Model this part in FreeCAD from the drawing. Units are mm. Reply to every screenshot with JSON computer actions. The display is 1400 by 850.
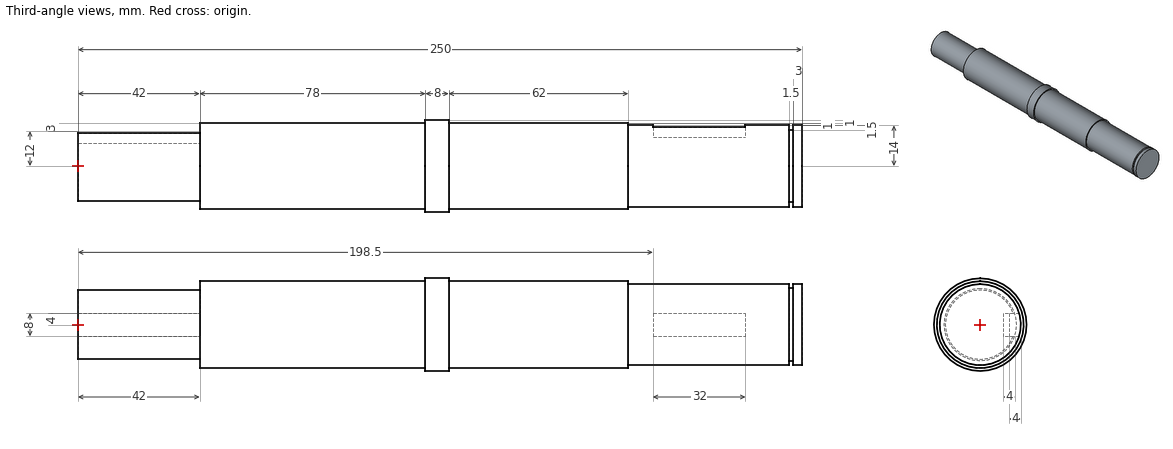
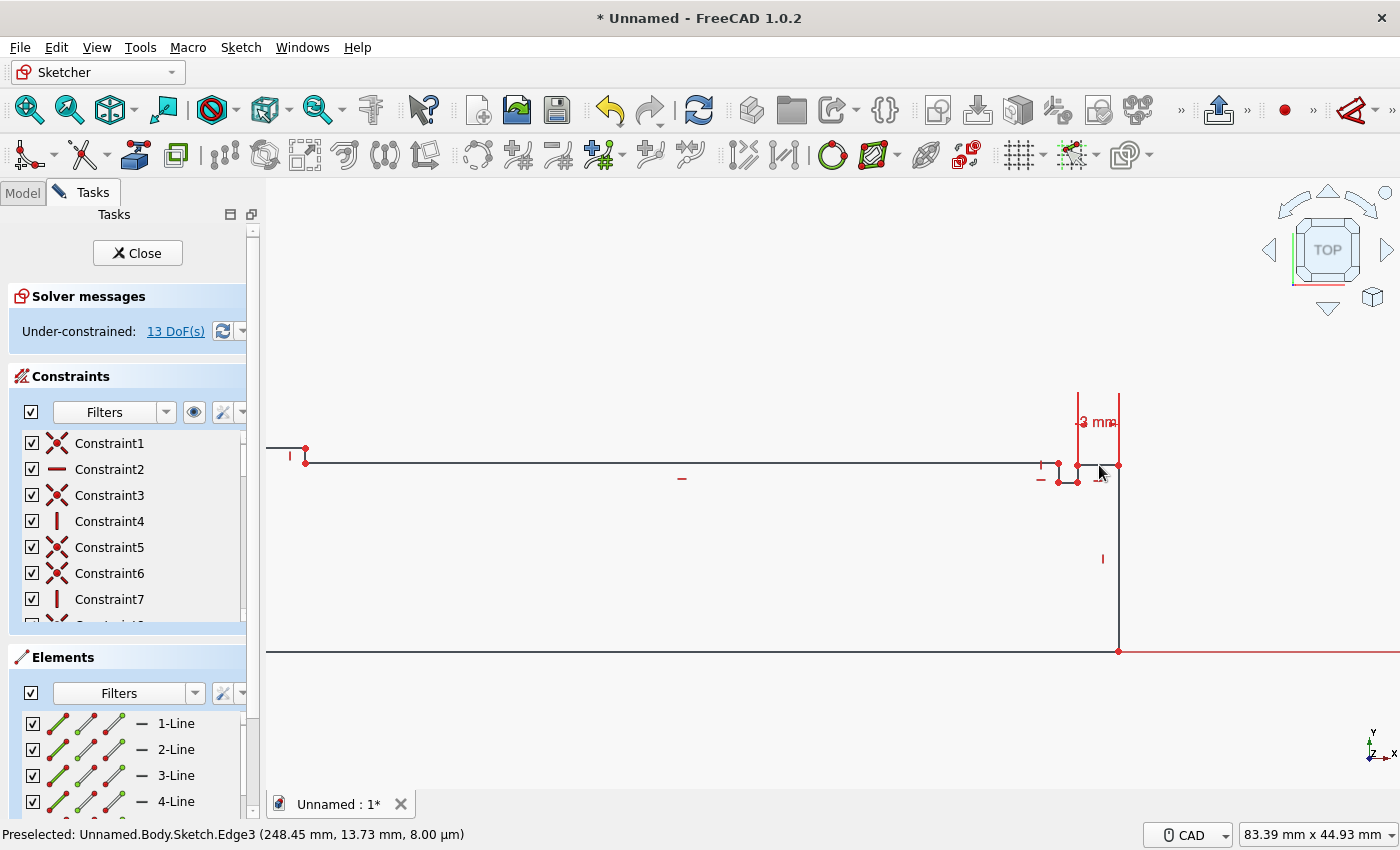
{"action": "scroll", "coordinate": [305, 456], "scroll_direction": "up", "scroll_amount": 6}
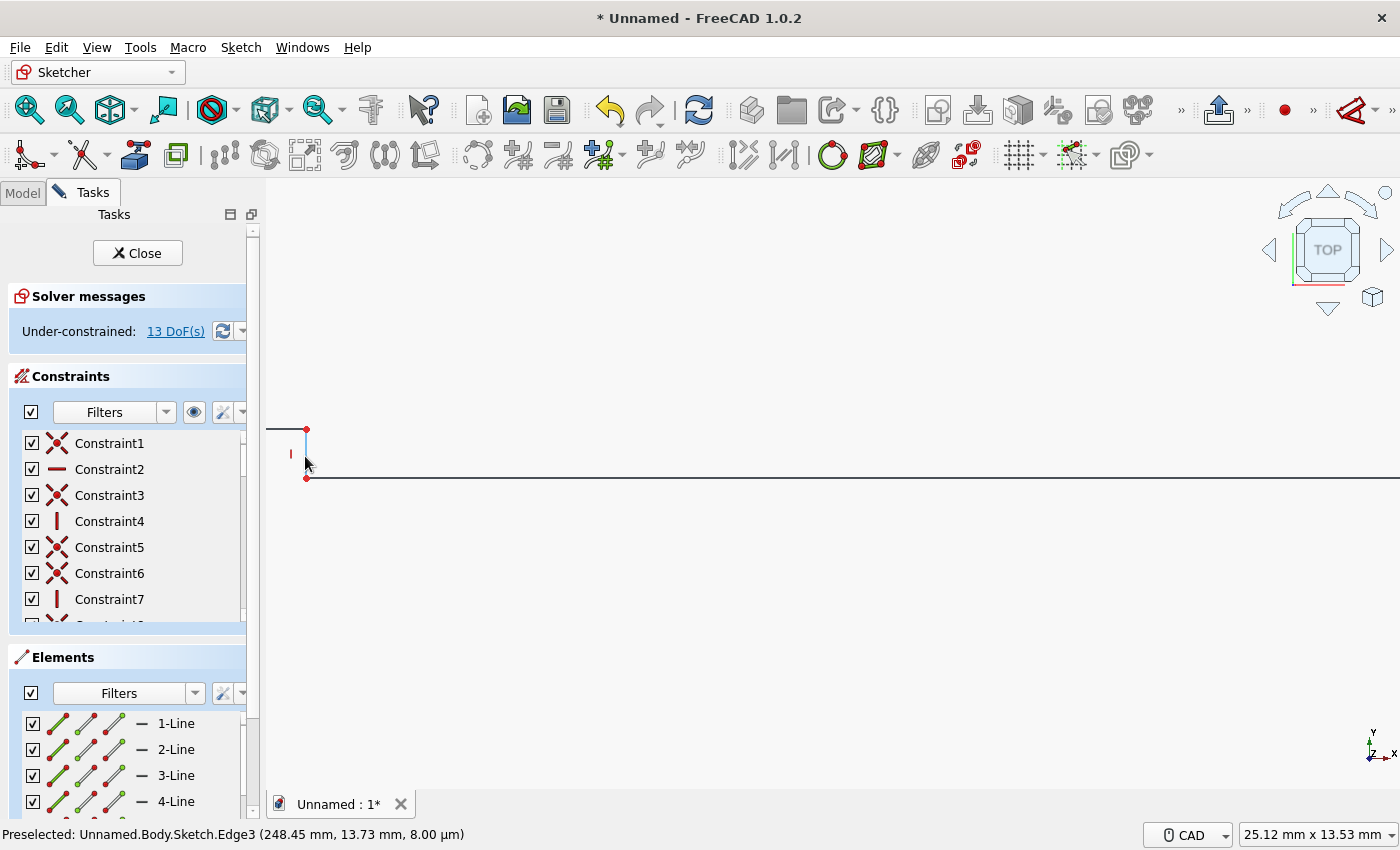
{"action": "left_click", "coordinate": [306, 454]}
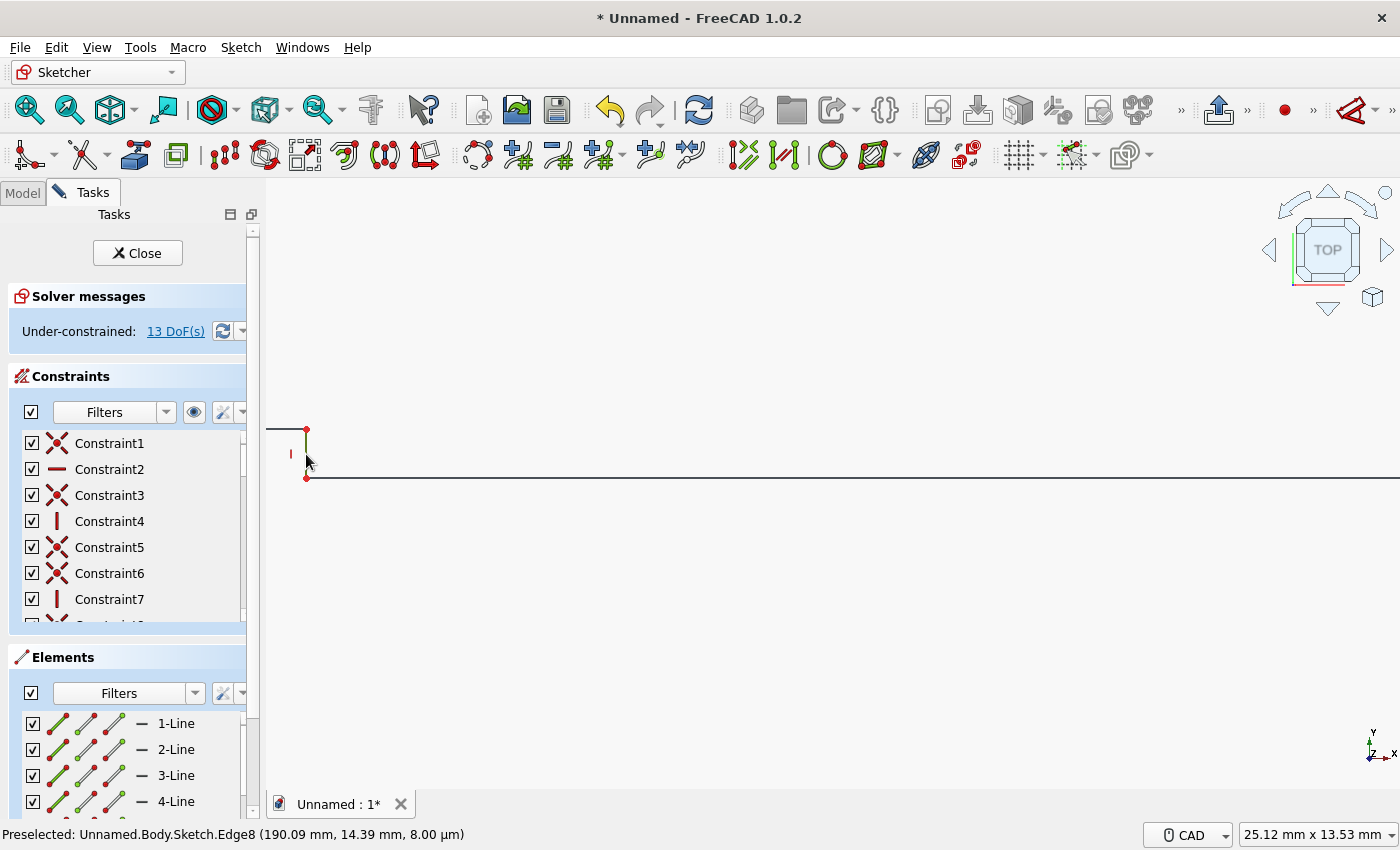
{"action": "left_click", "coordinate": [1378, 110]}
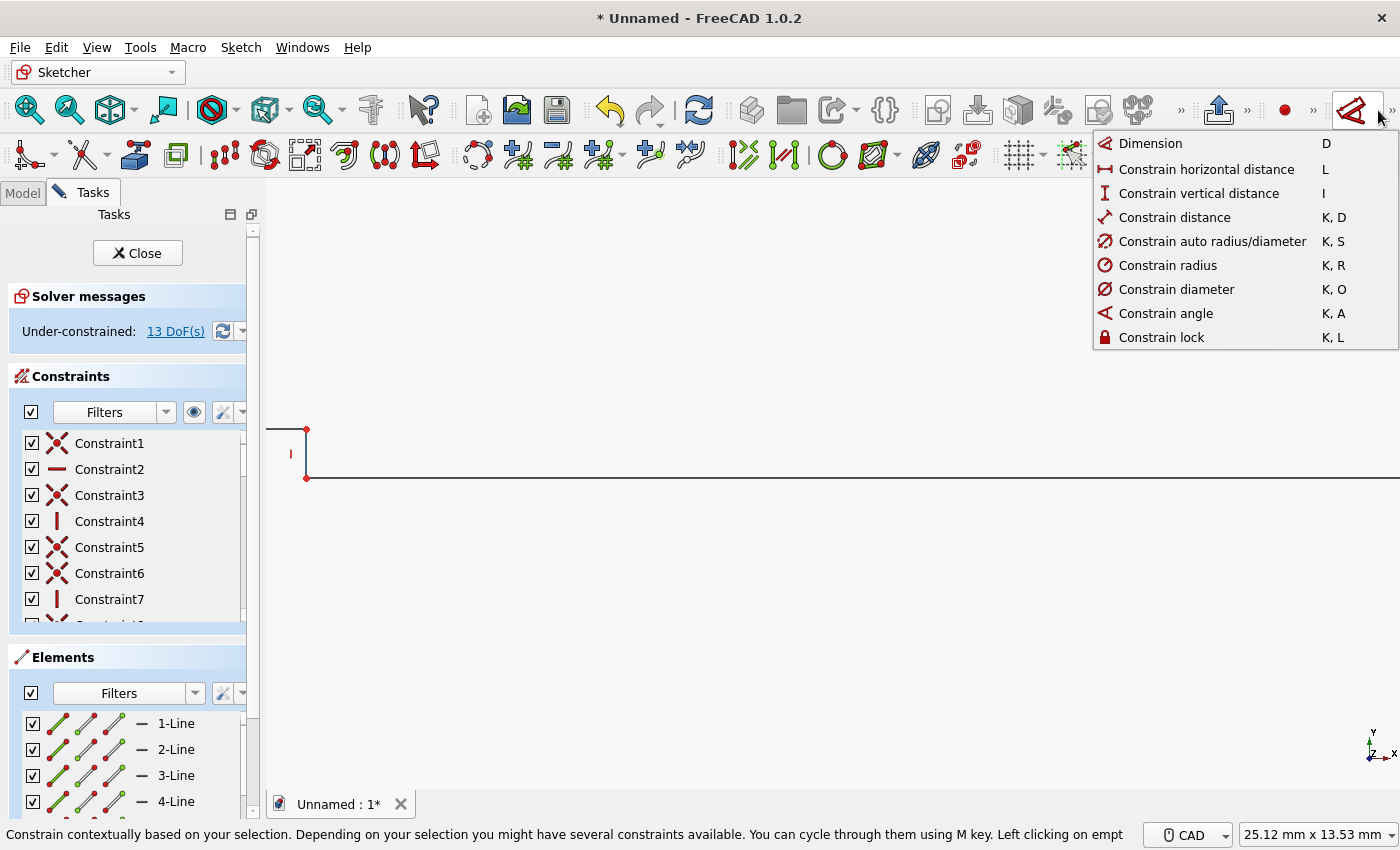
{"action": "left_click", "coordinate": [1246, 193]}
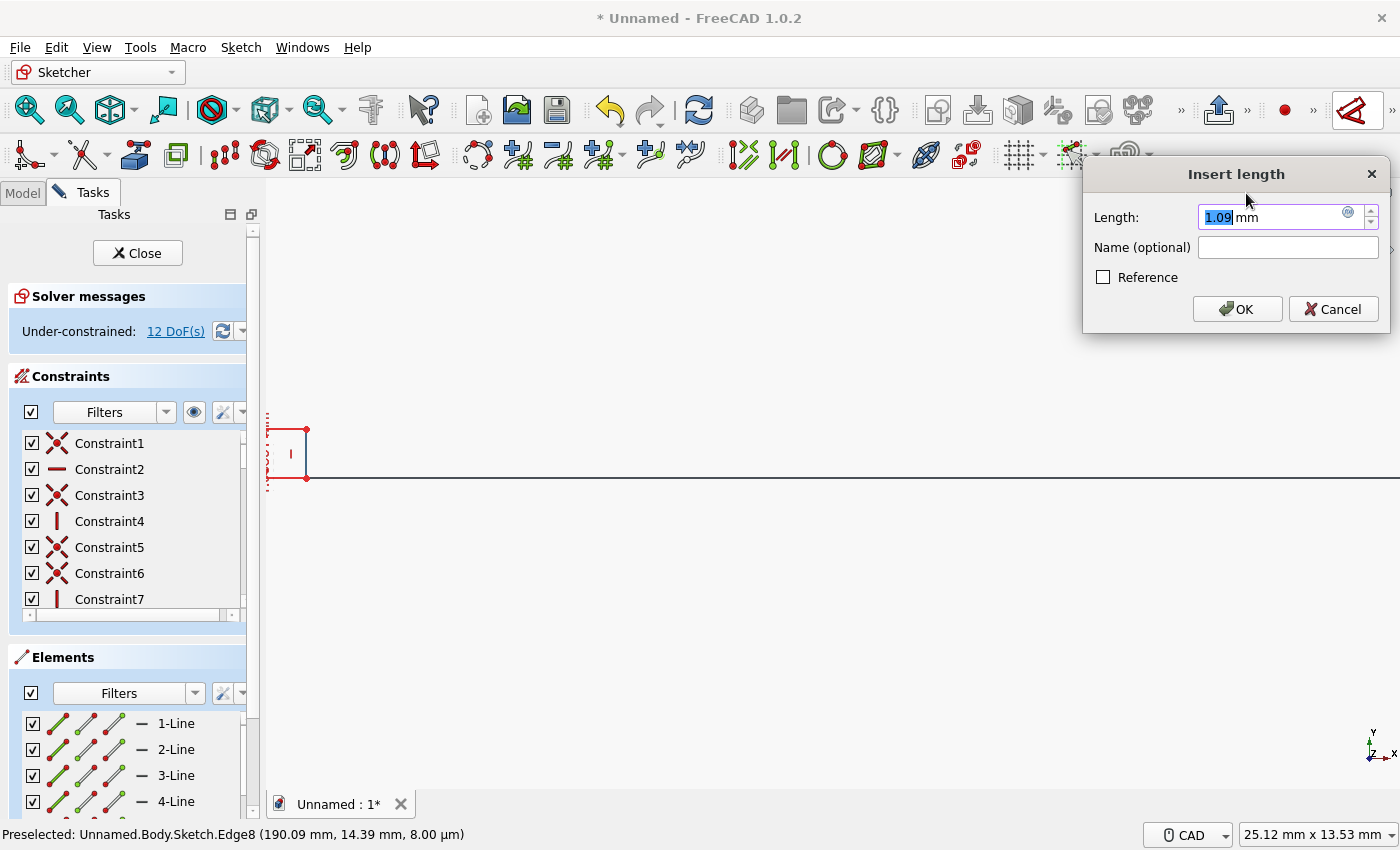
{"action": "type", "text": "1"}
{"action": "key", "text": "Return"}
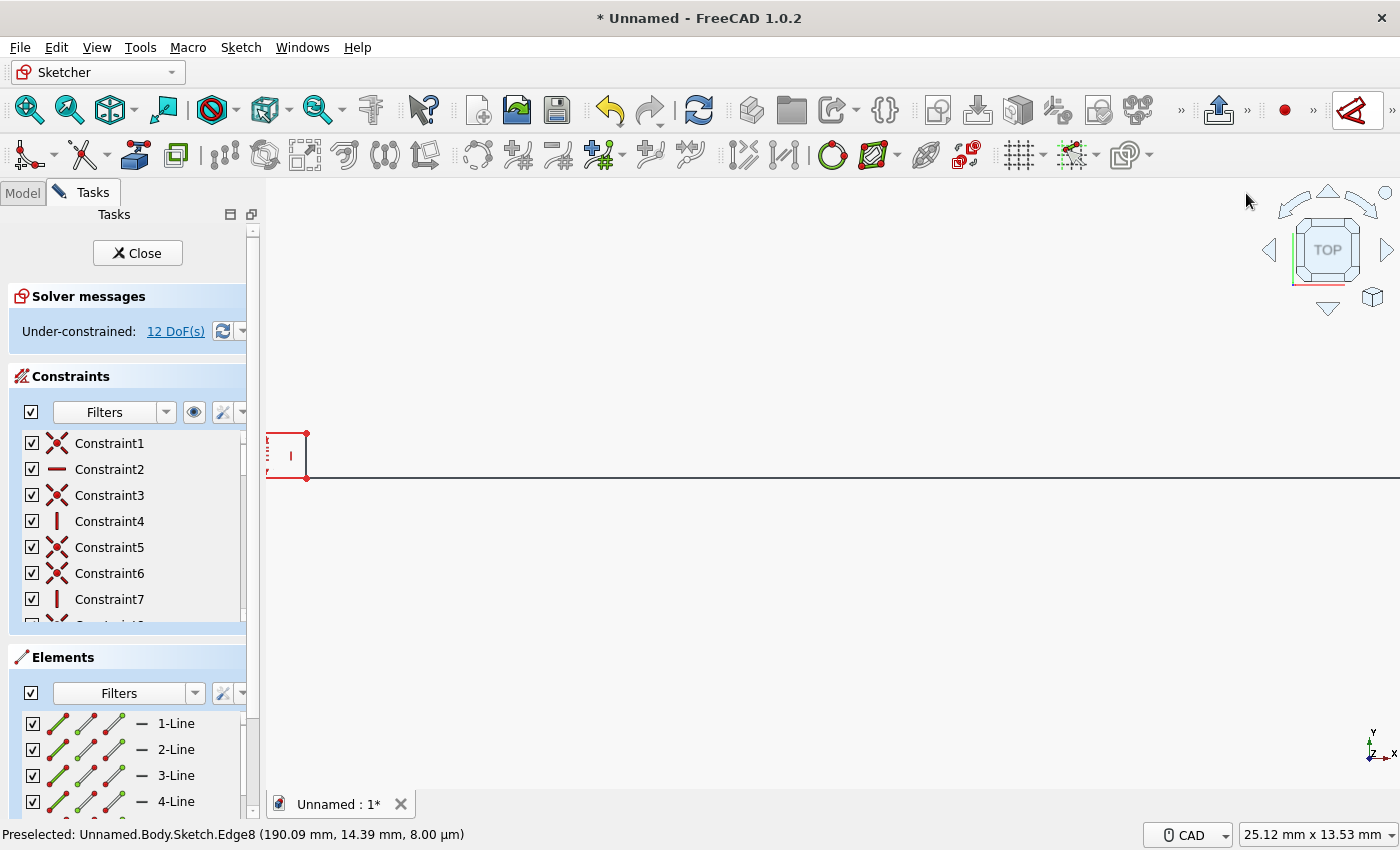
{"action": "scroll", "coordinate": [984, 467], "scroll_direction": "down", "scroll_amount": 14}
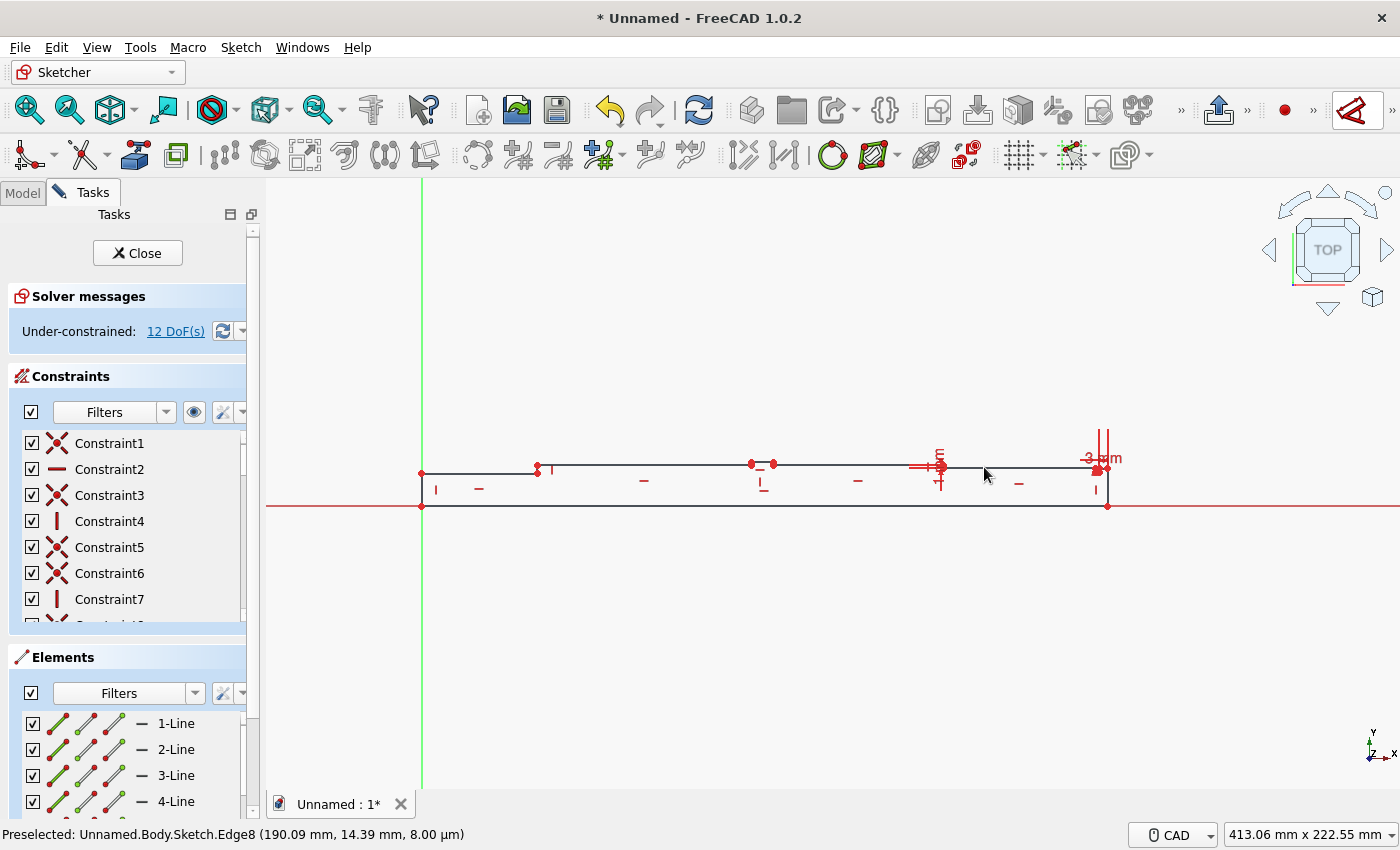
{"action": "scroll", "coordinate": [773, 465], "scroll_direction": "up", "scroll_amount": 14}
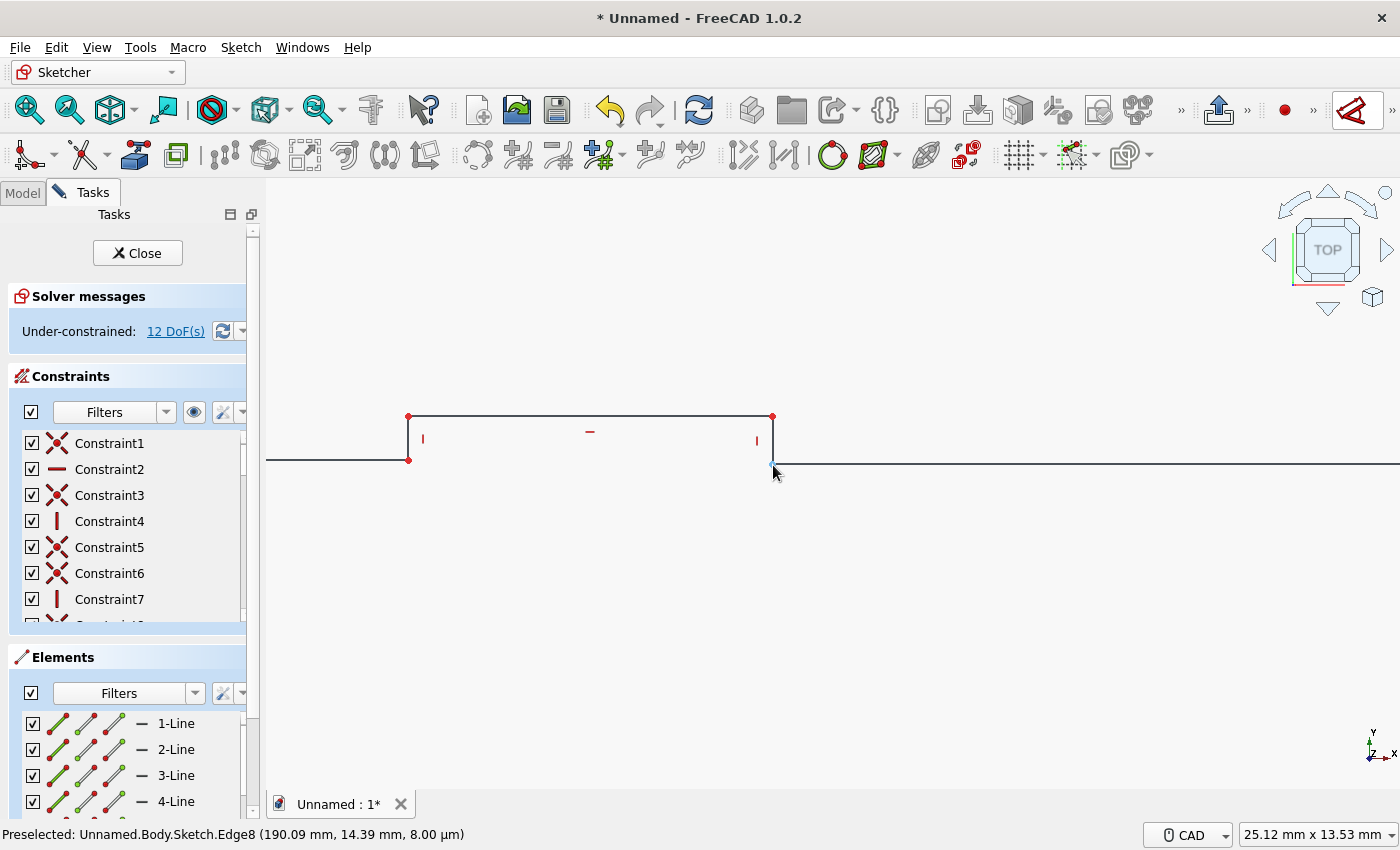
{"action": "left_click", "coordinate": [773, 450]}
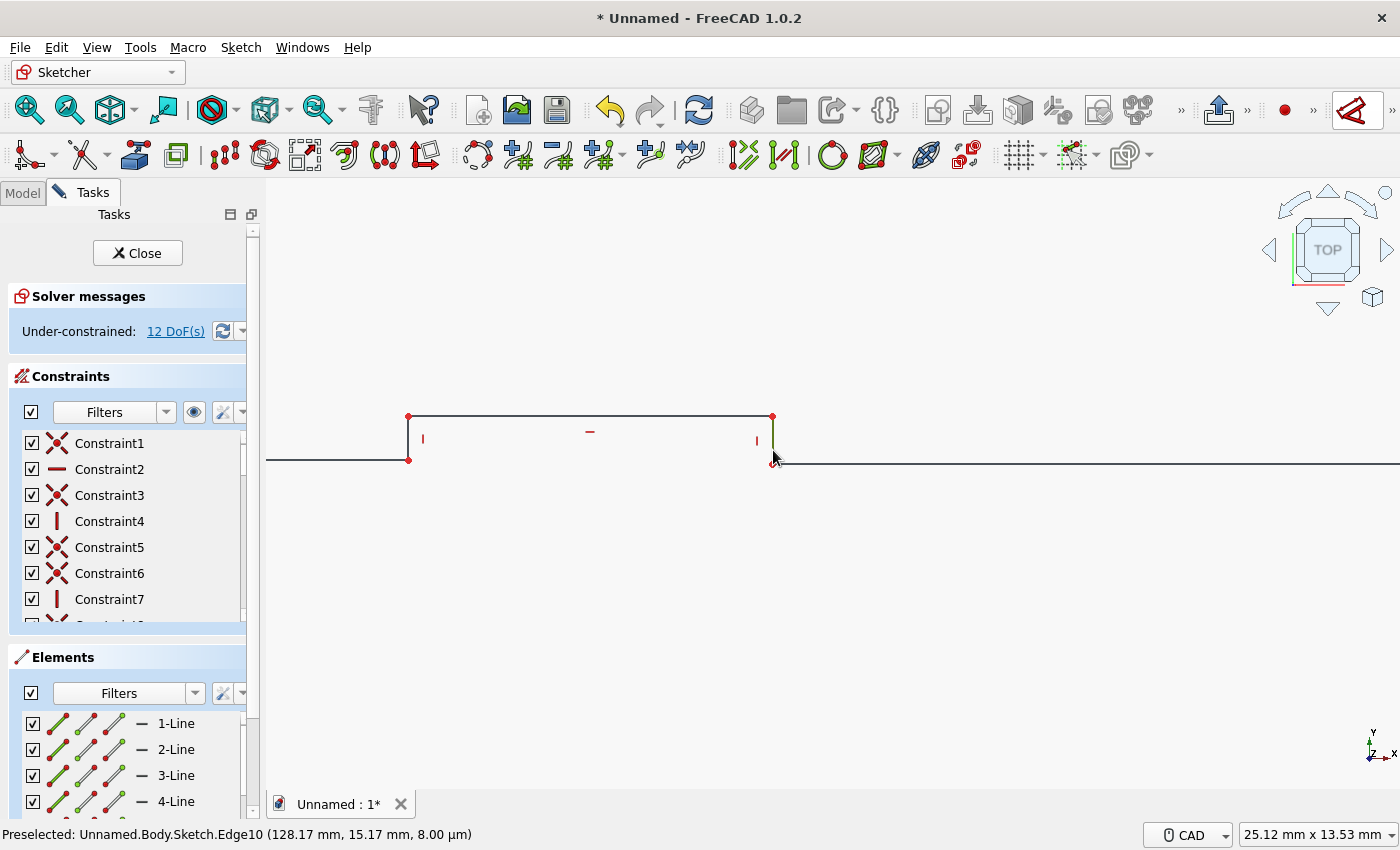
{"action": "left_click", "coordinate": [1378, 110]}